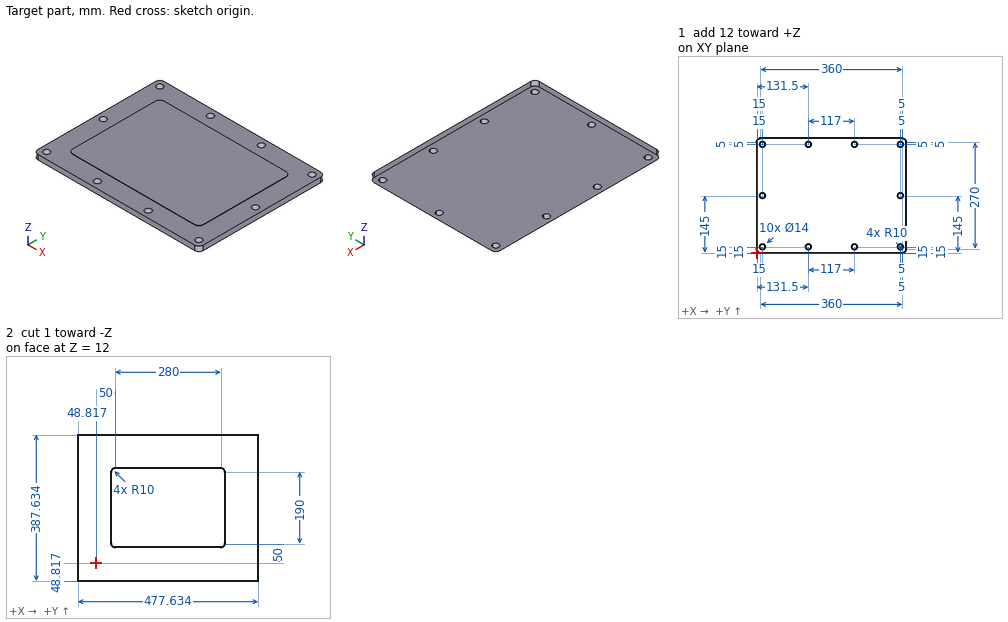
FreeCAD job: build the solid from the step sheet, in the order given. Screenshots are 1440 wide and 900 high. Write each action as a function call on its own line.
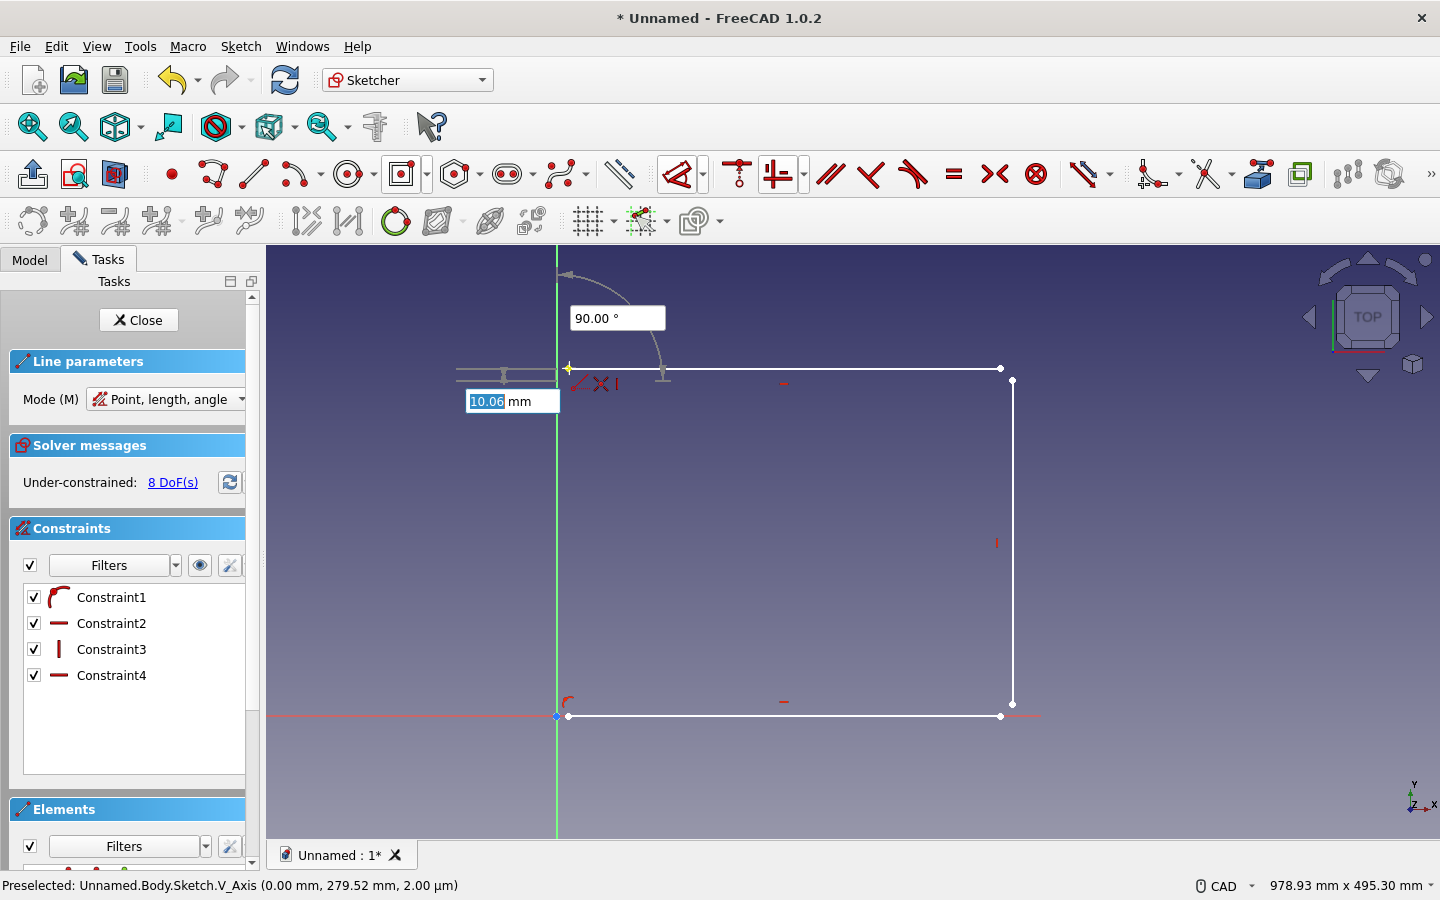
scroll(557, 704, up, 2)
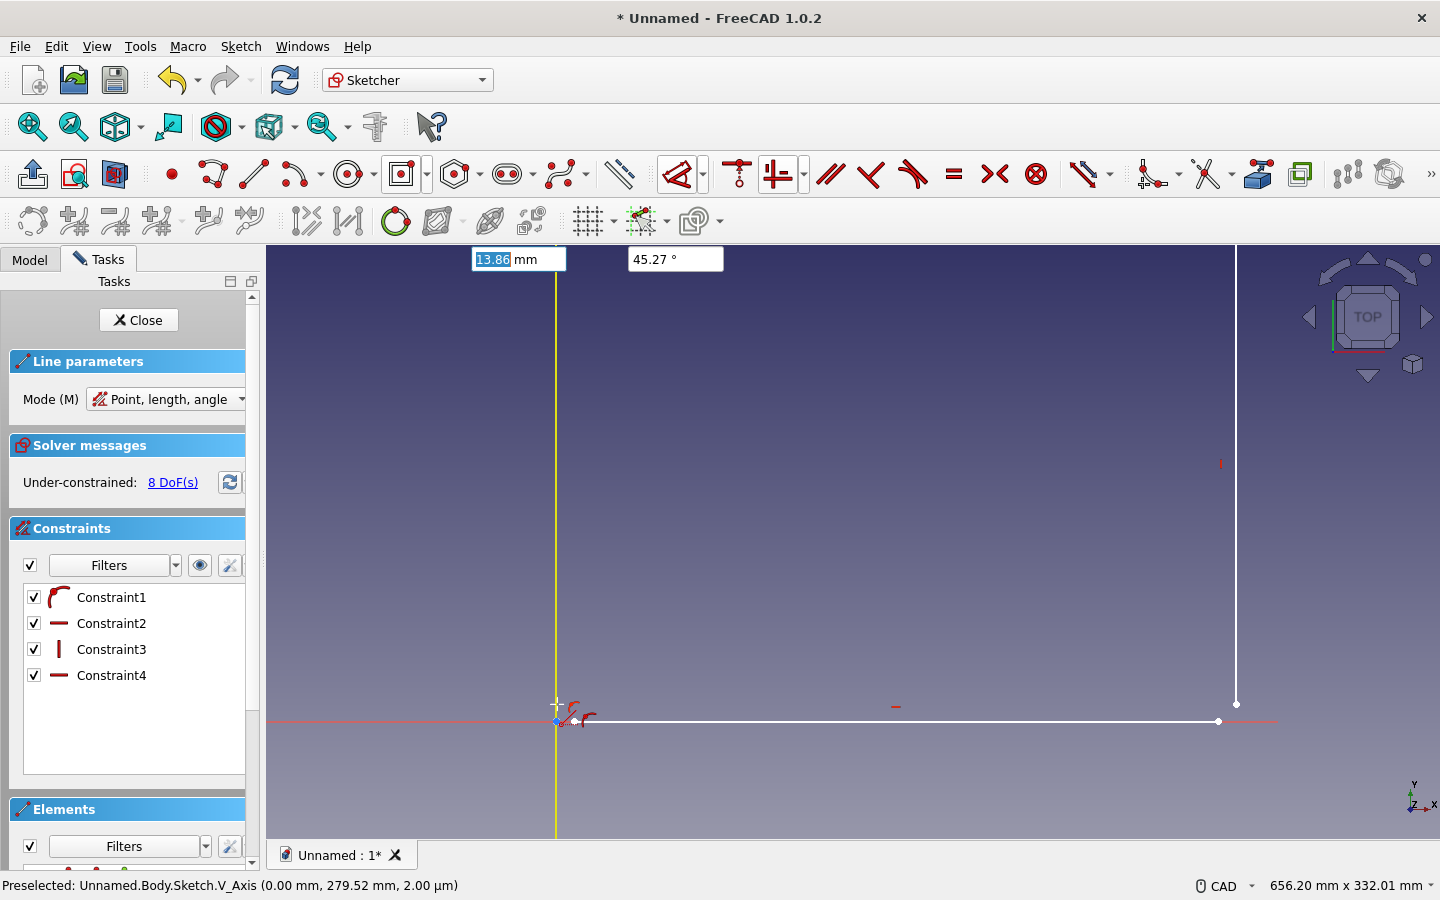
click(565, 704)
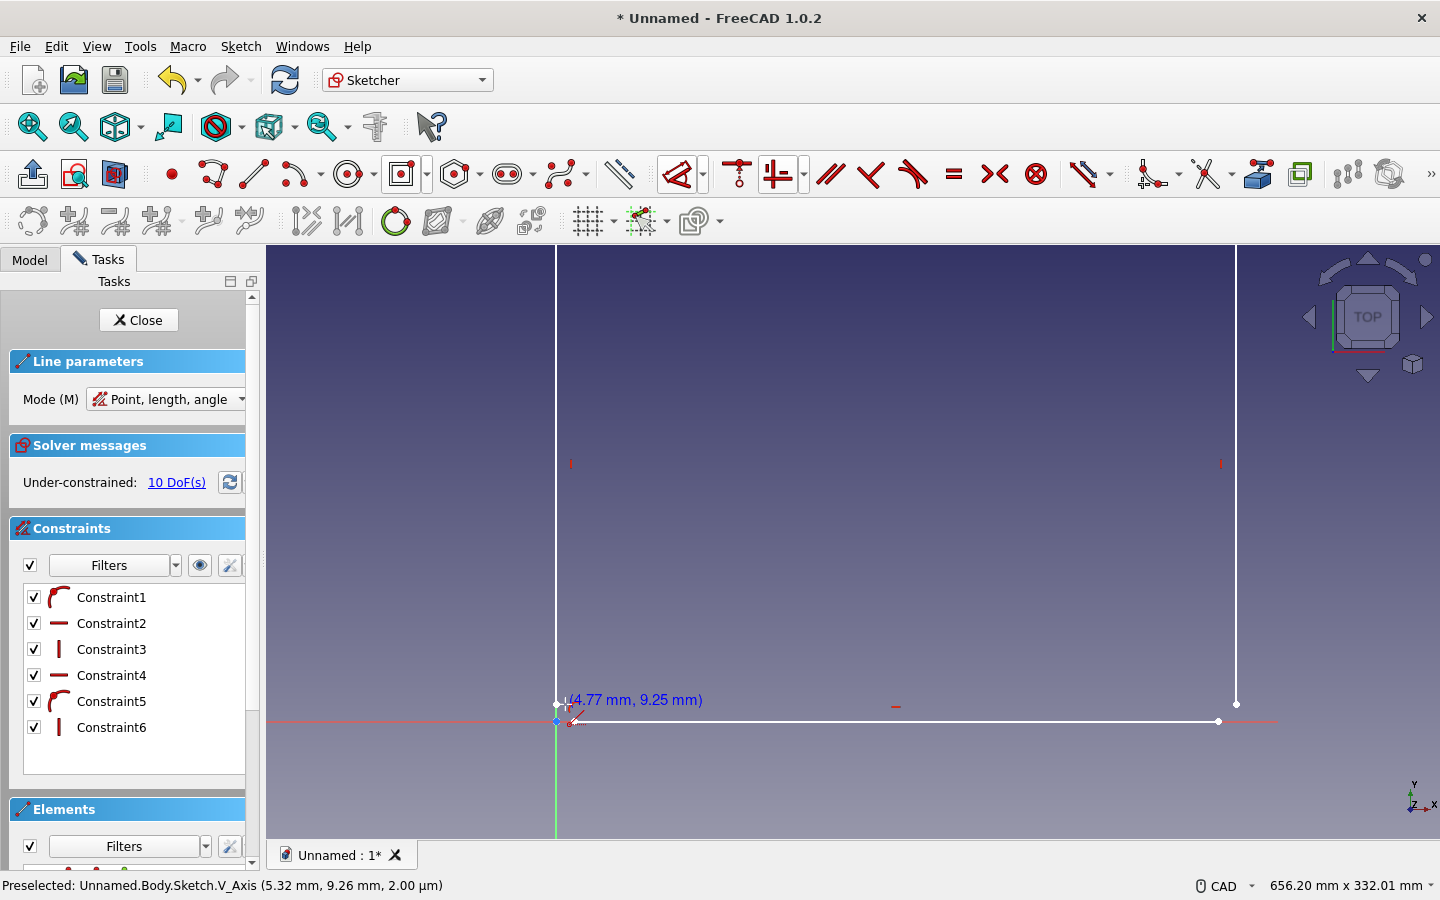
click(320, 174)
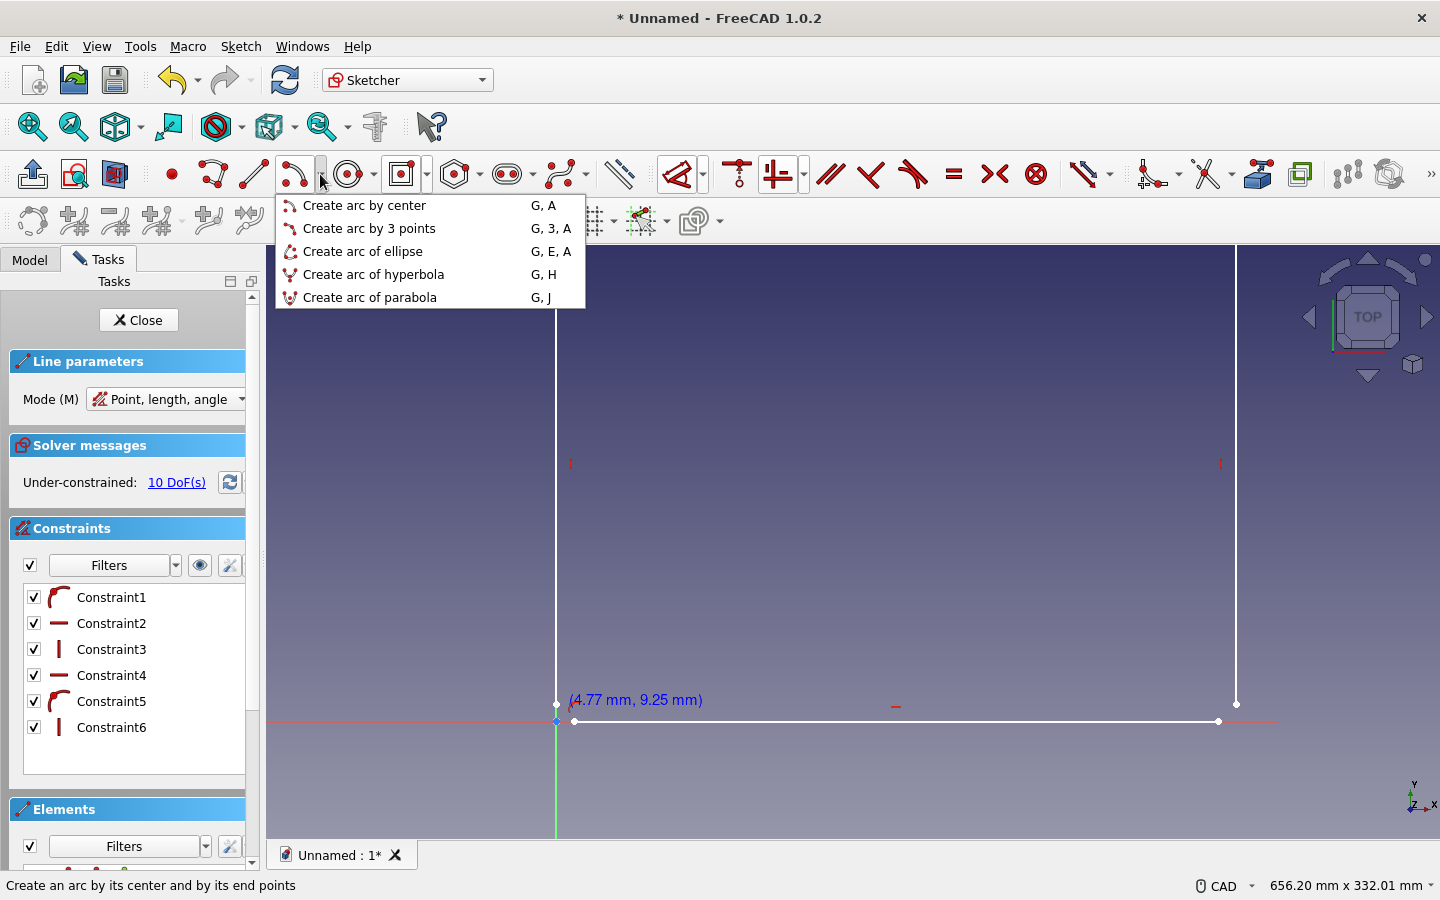
click(430, 228)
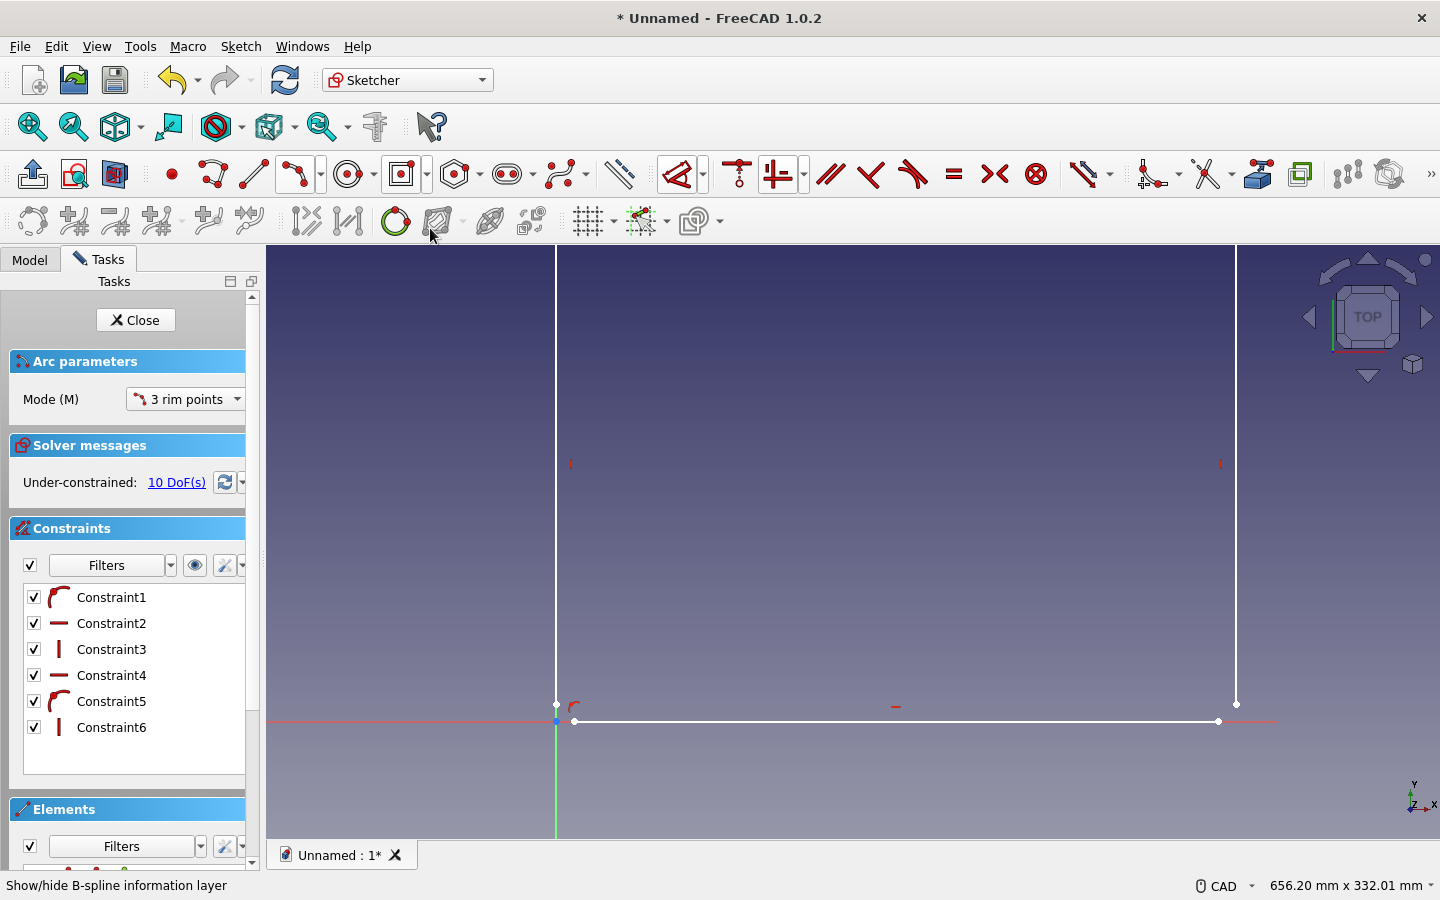
click(1218, 712)
click(1236, 704)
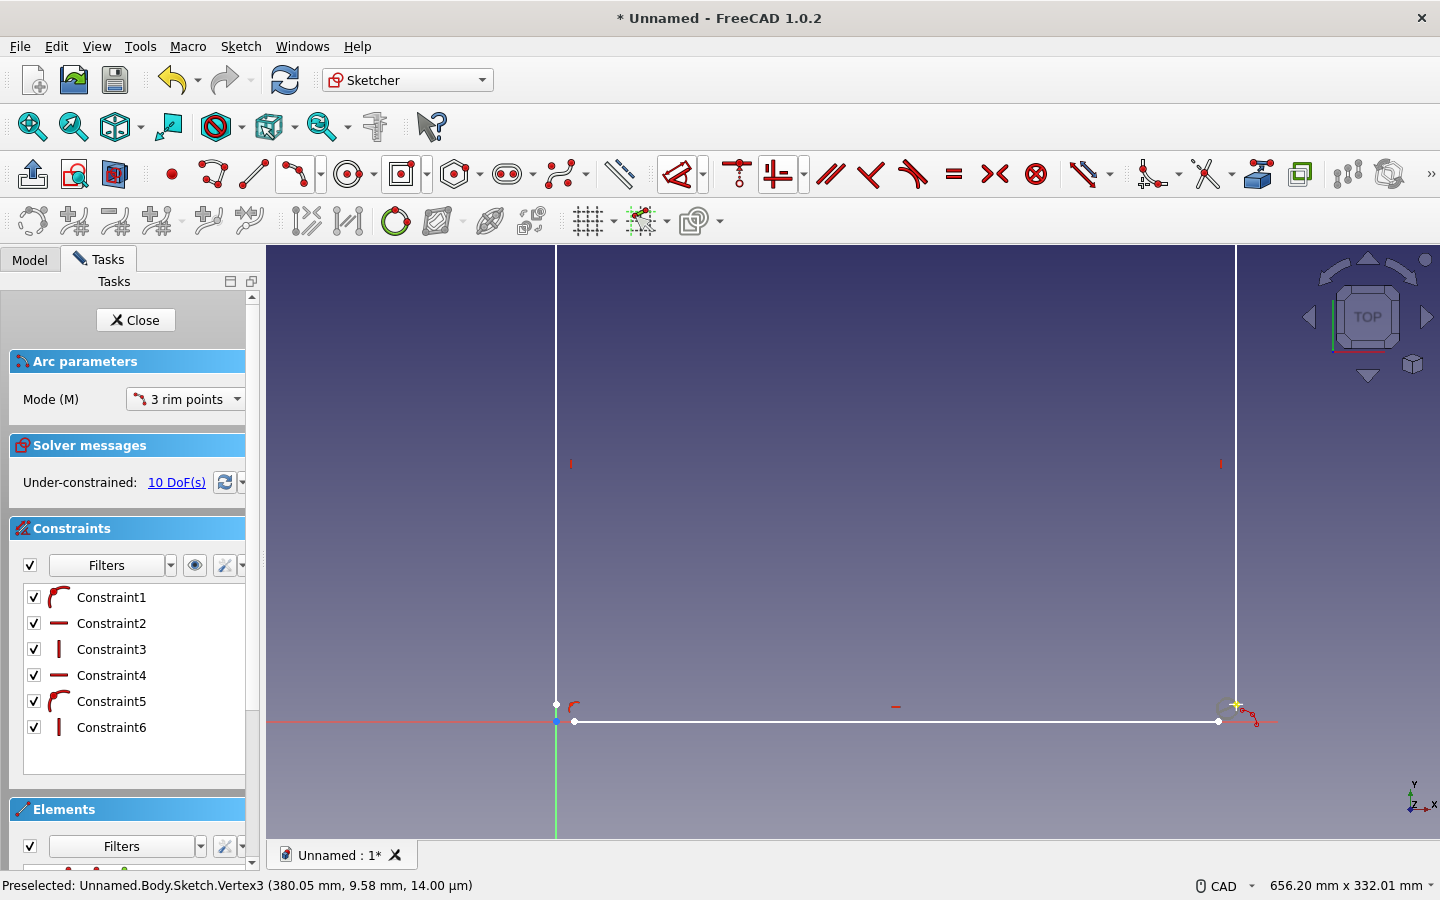
scroll(1231, 716, up, 6)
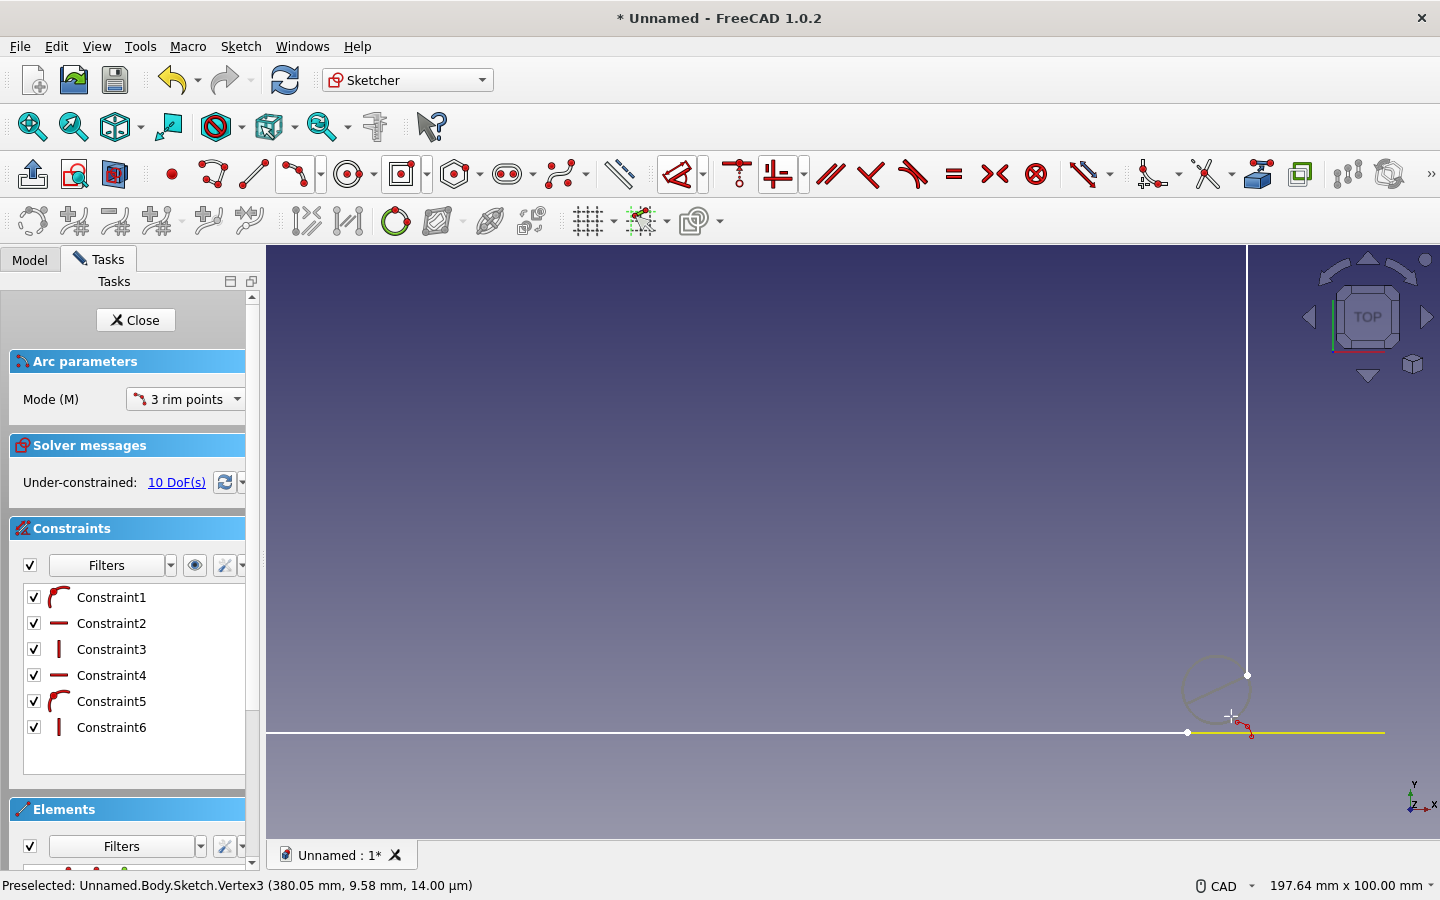
click(1229, 715)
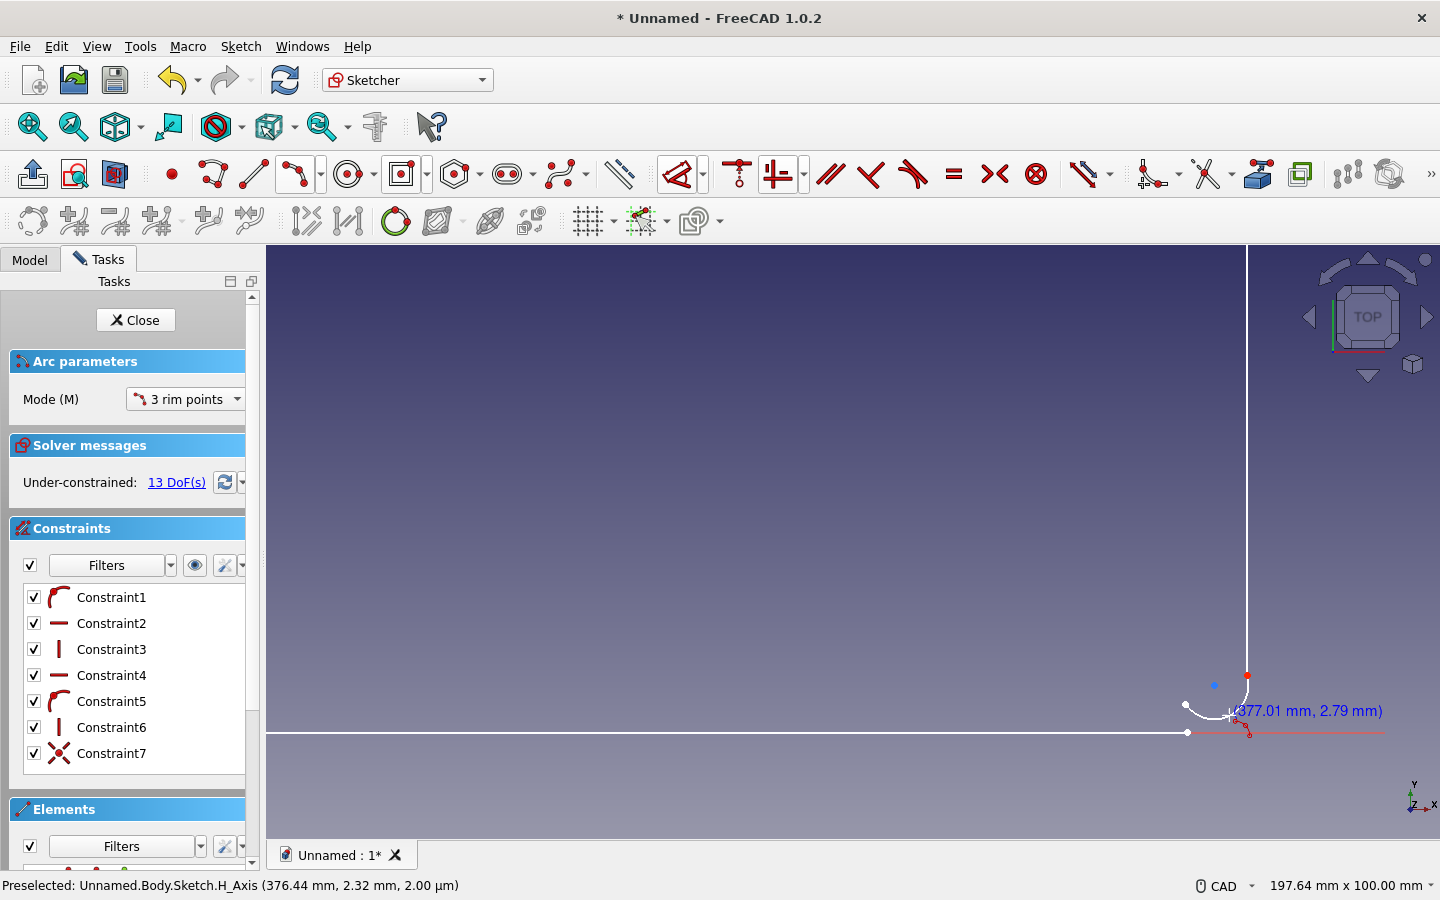
scroll(953, 712, down, 8)